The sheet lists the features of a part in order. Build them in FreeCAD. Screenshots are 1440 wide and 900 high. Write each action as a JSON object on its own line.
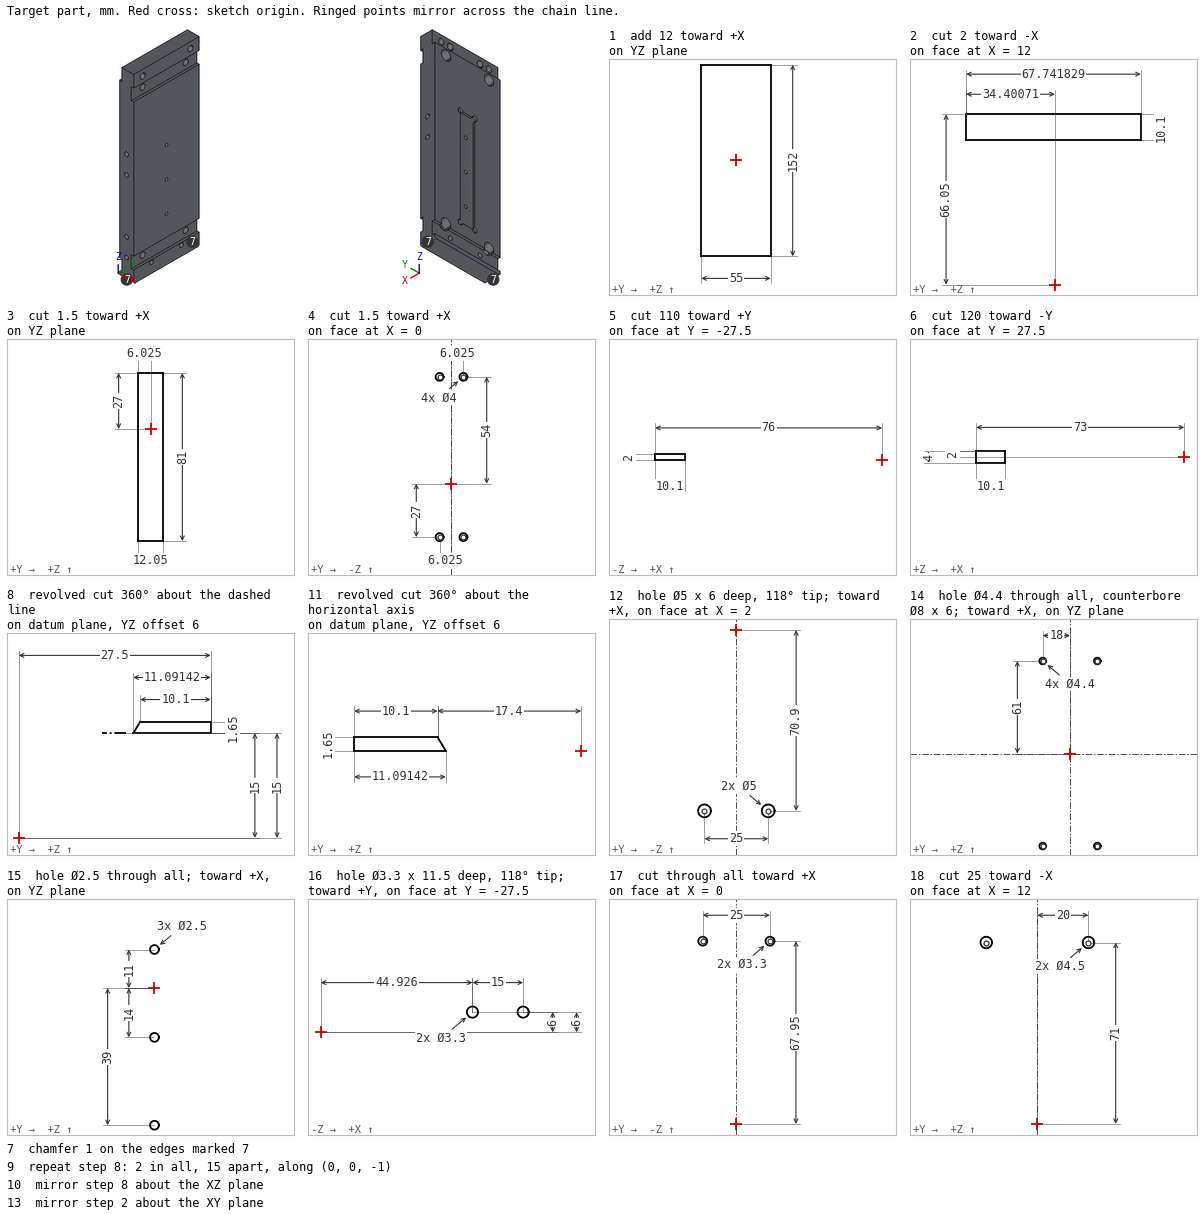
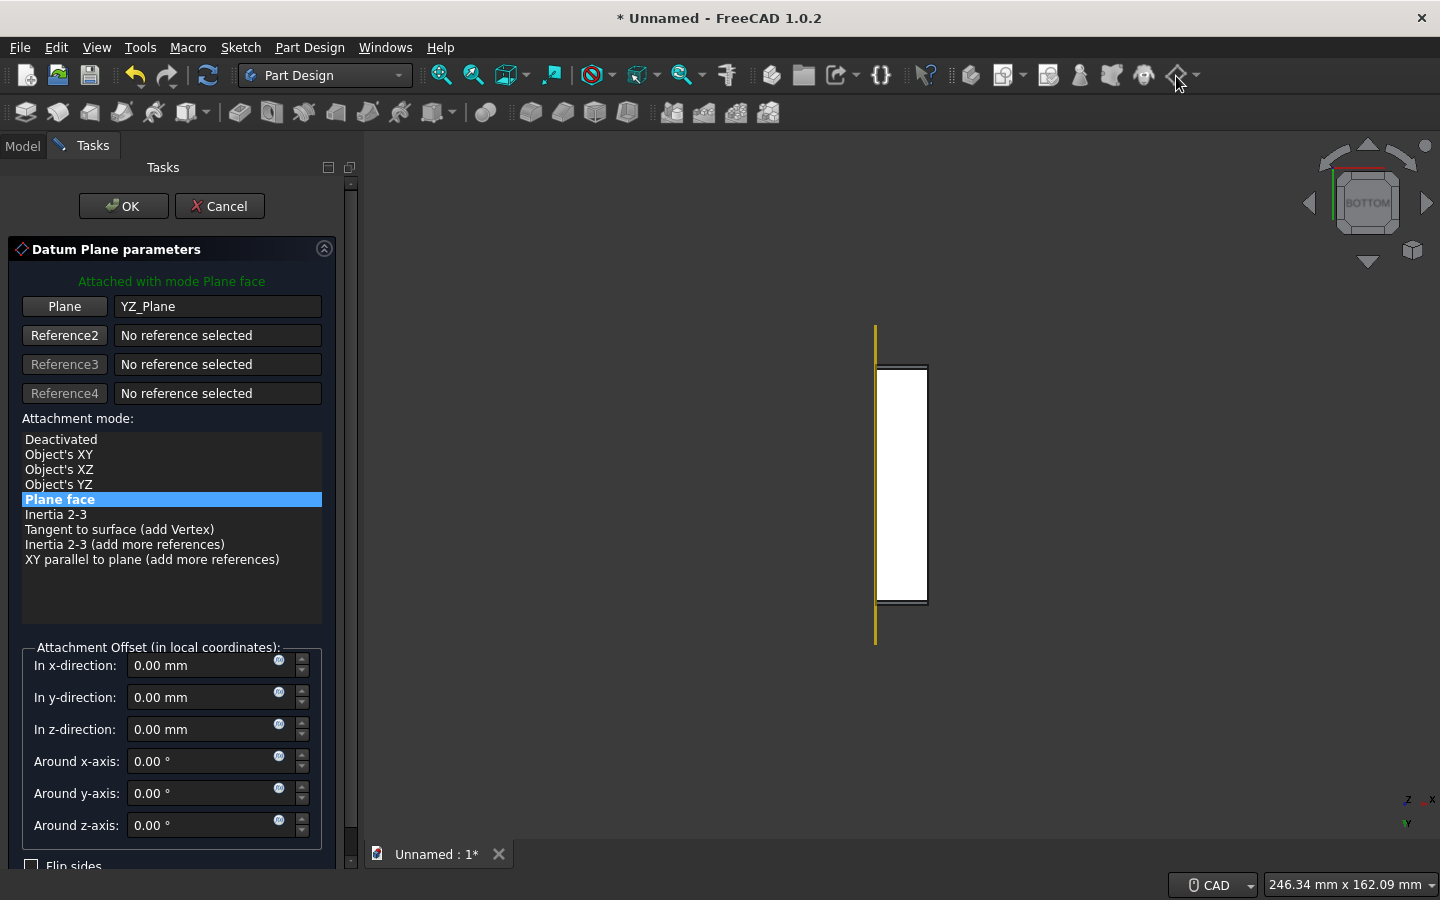
{"action": "triple_click", "coordinate": [210, 729]}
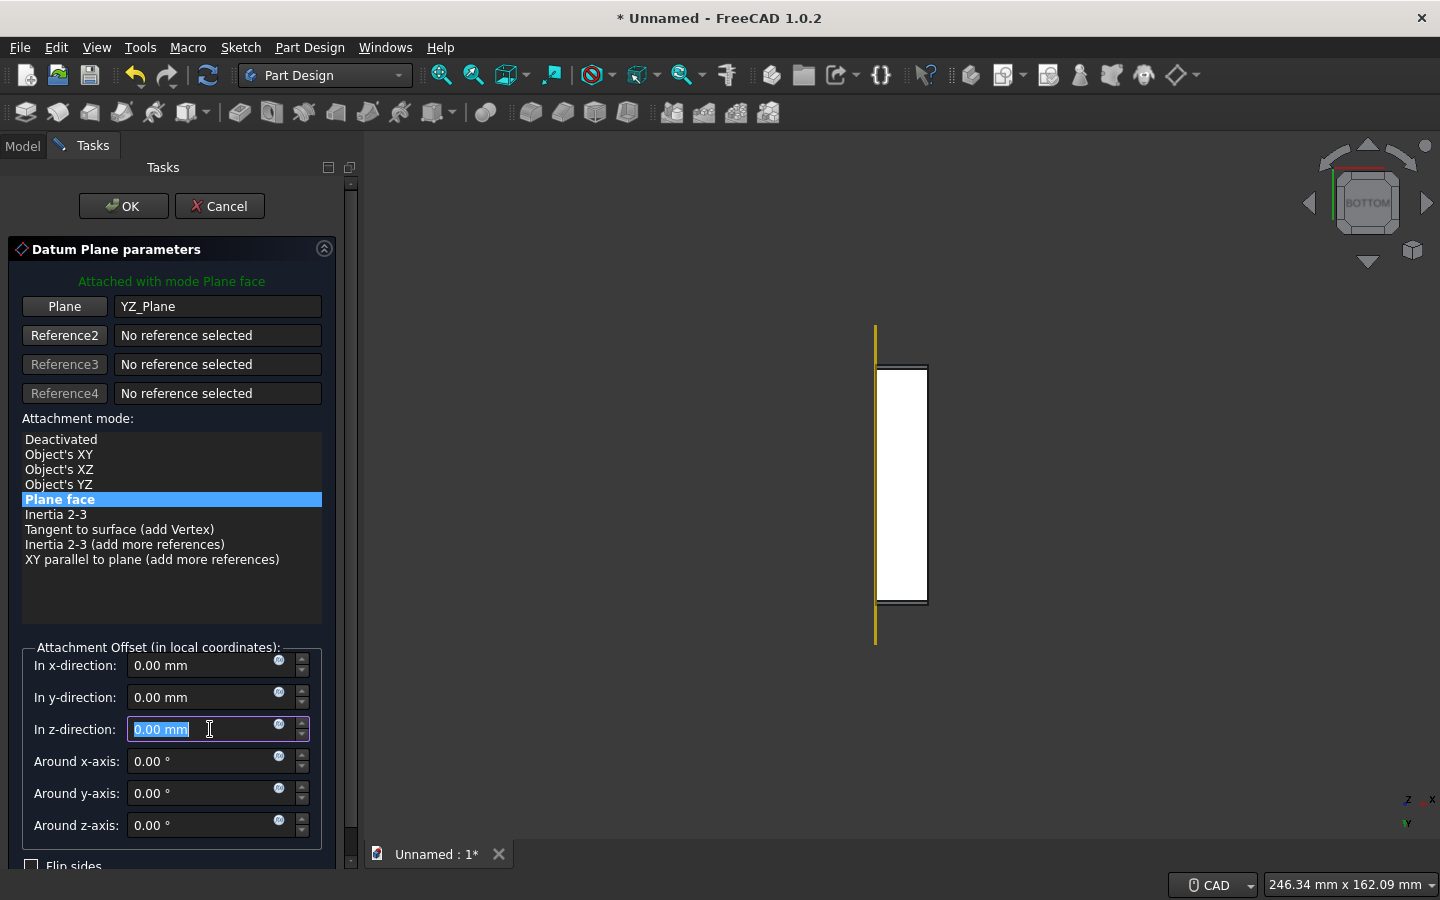
{"action": "type", "text": "6"}
{"action": "key", "text": "Tab"}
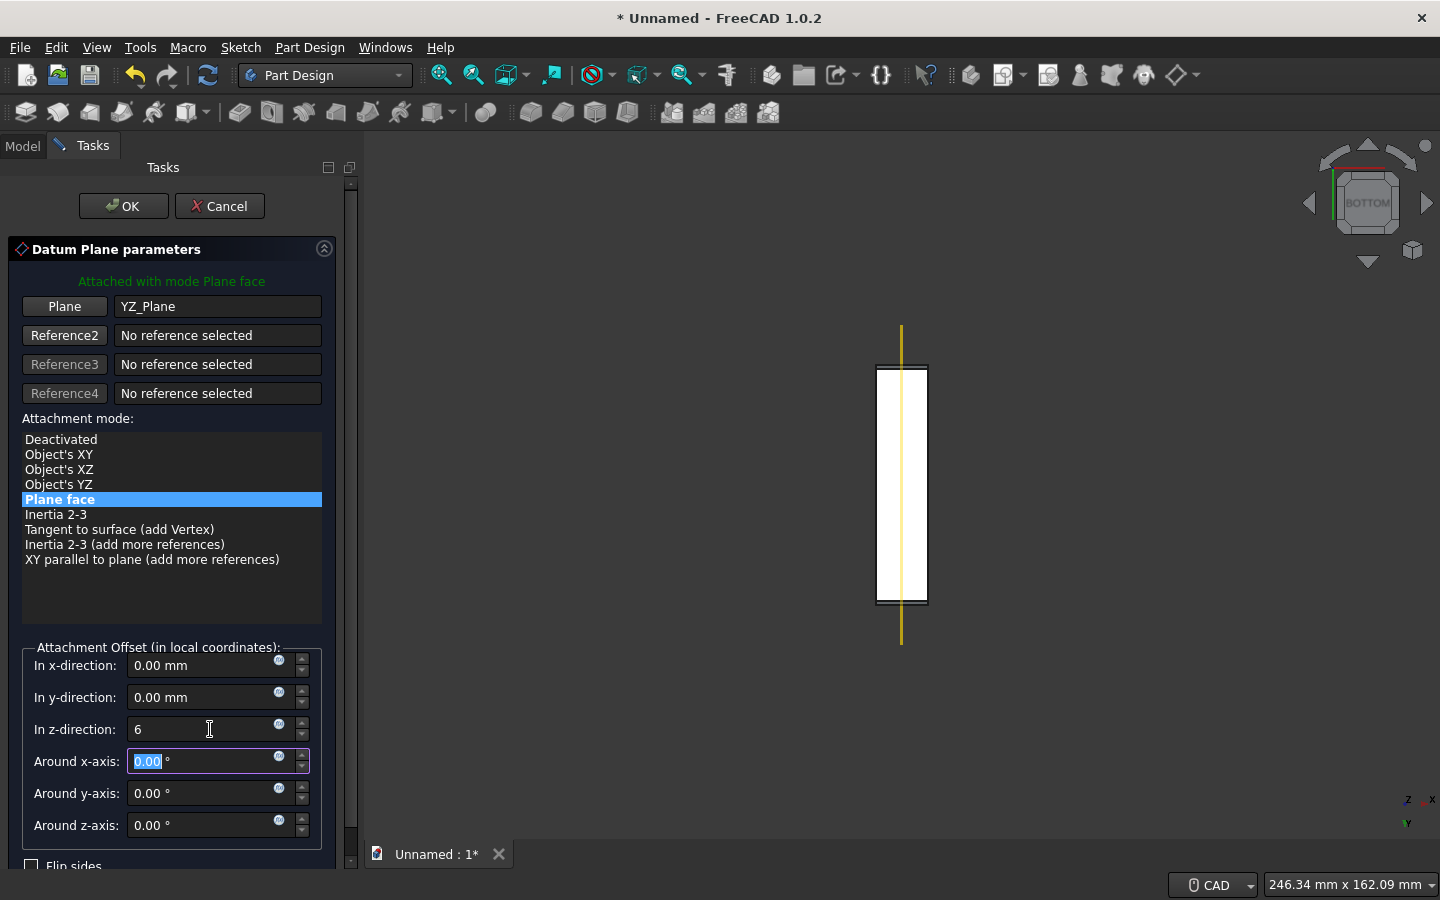
{"action": "left_click", "coordinate": [124, 206]}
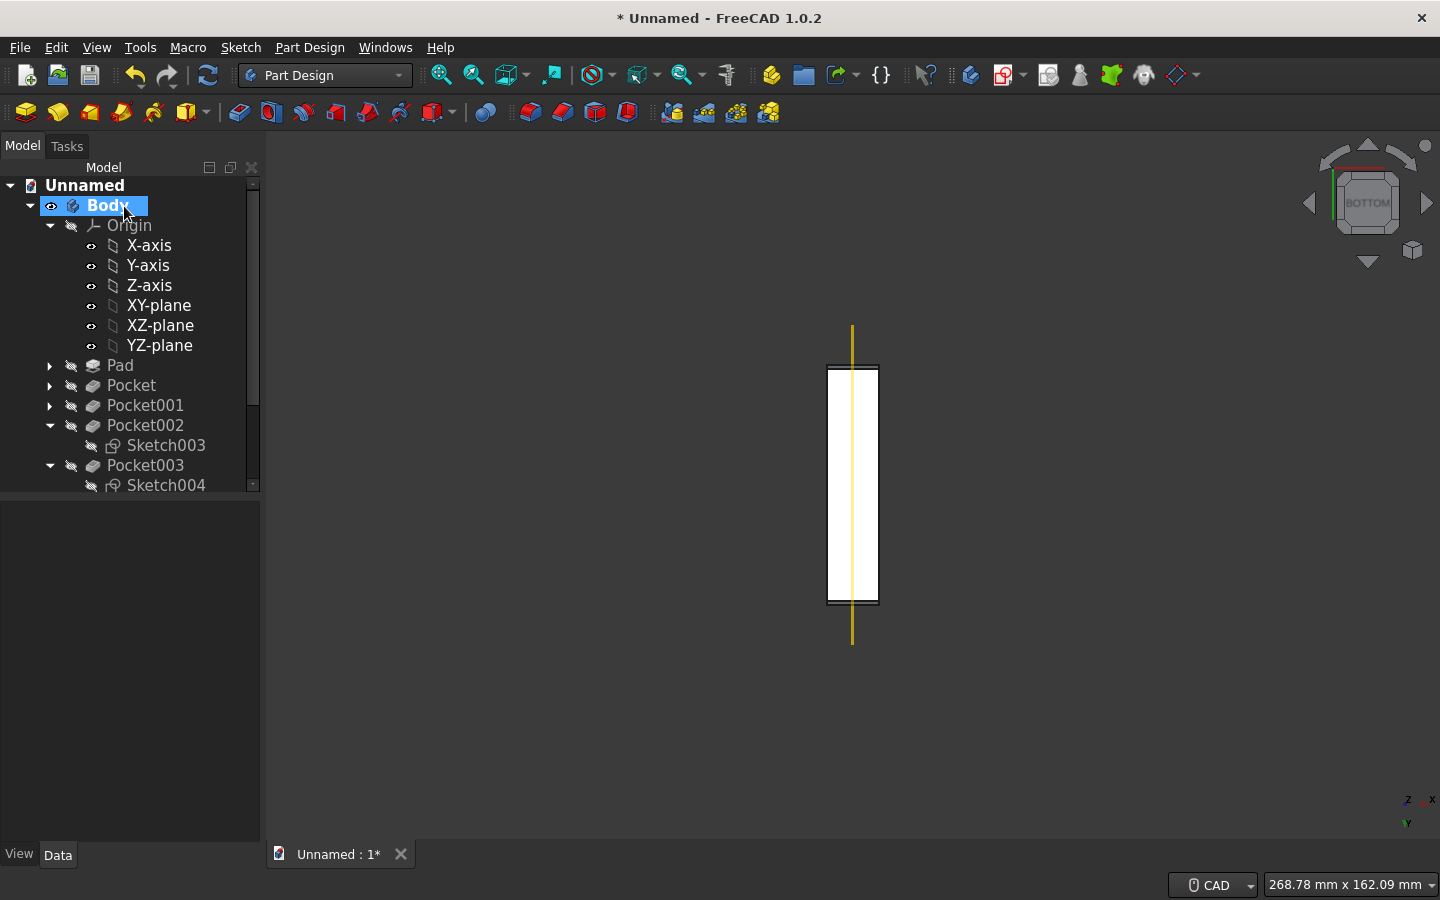
{"action": "scroll", "coordinate": [100, 341], "scroll_direction": "down", "scroll_amount": 3}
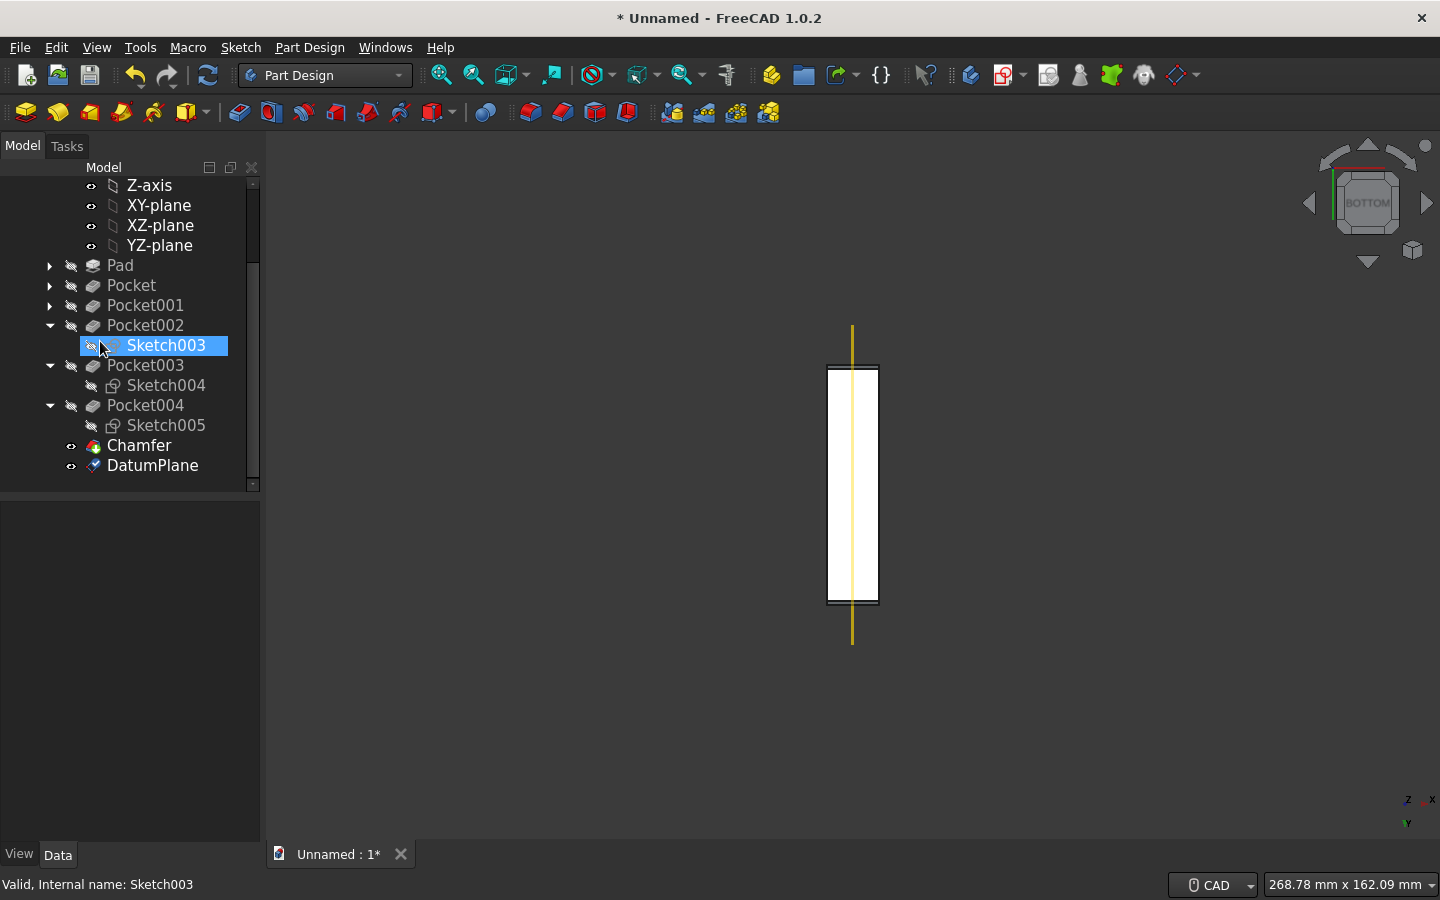
{"action": "left_click", "coordinate": [116, 466]}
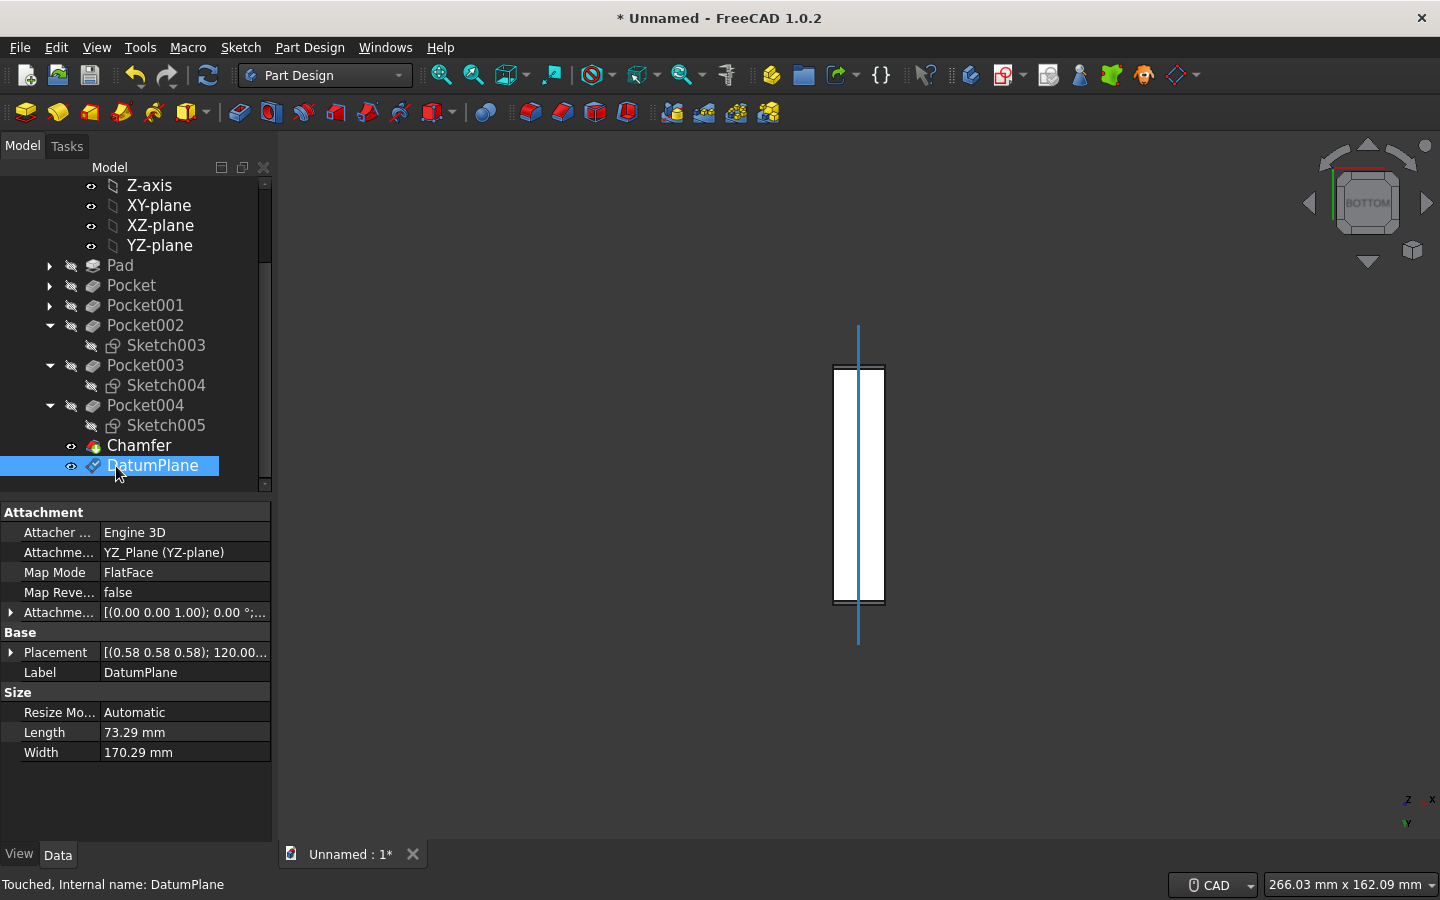
{"action": "left_click", "coordinate": [1004, 76]}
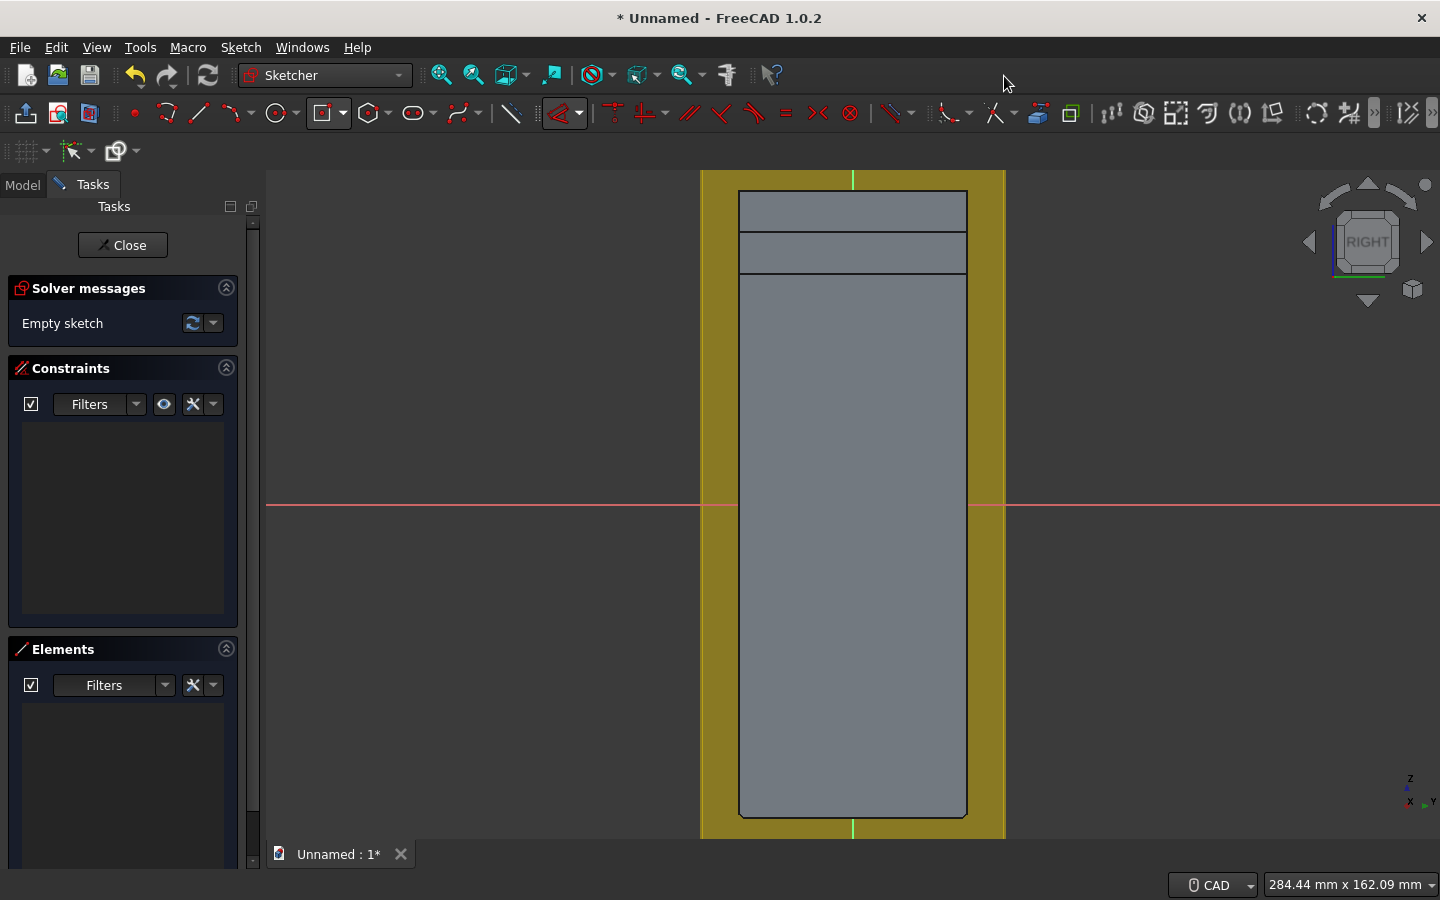
{"action": "left_click", "coordinate": [90, 114]}